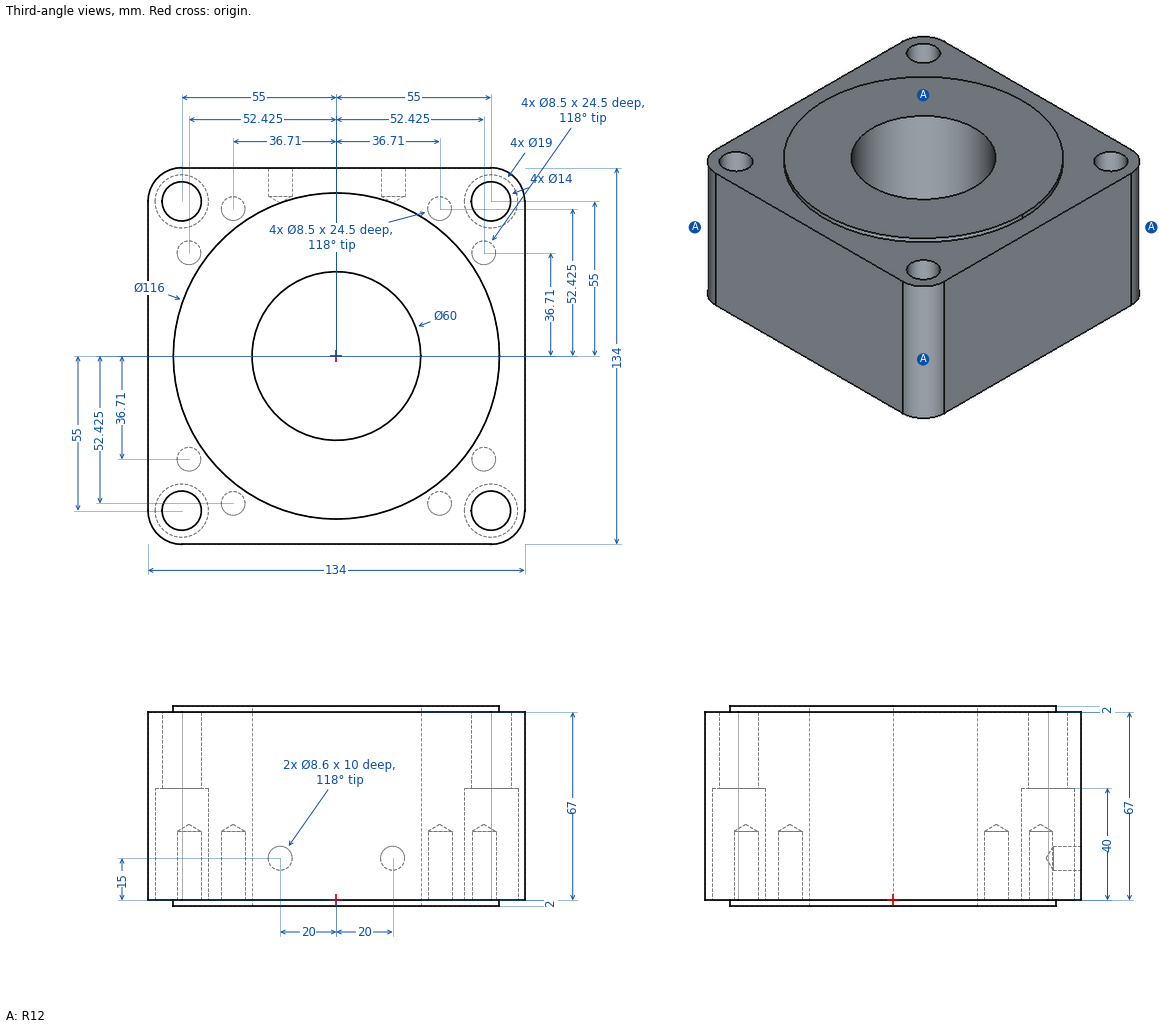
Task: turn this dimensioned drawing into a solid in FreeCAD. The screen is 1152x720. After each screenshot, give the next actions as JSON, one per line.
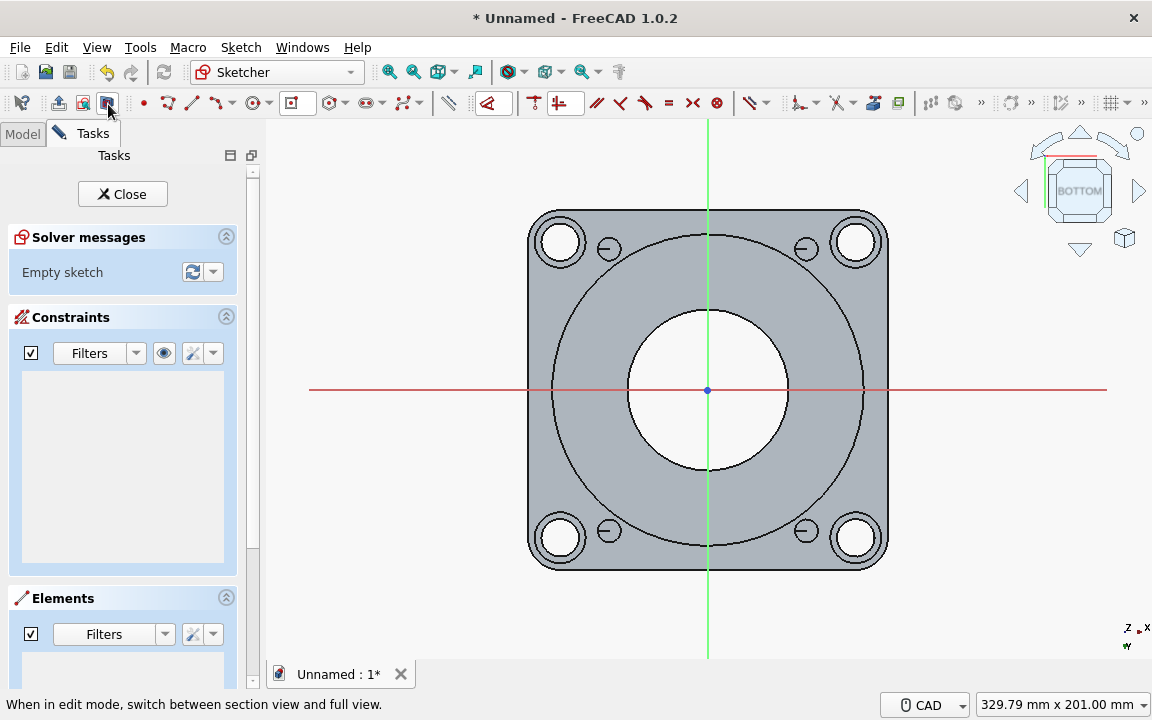
{"action": "scroll", "coordinate": [845, 392], "scroll_direction": "up", "scroll_amount": 2}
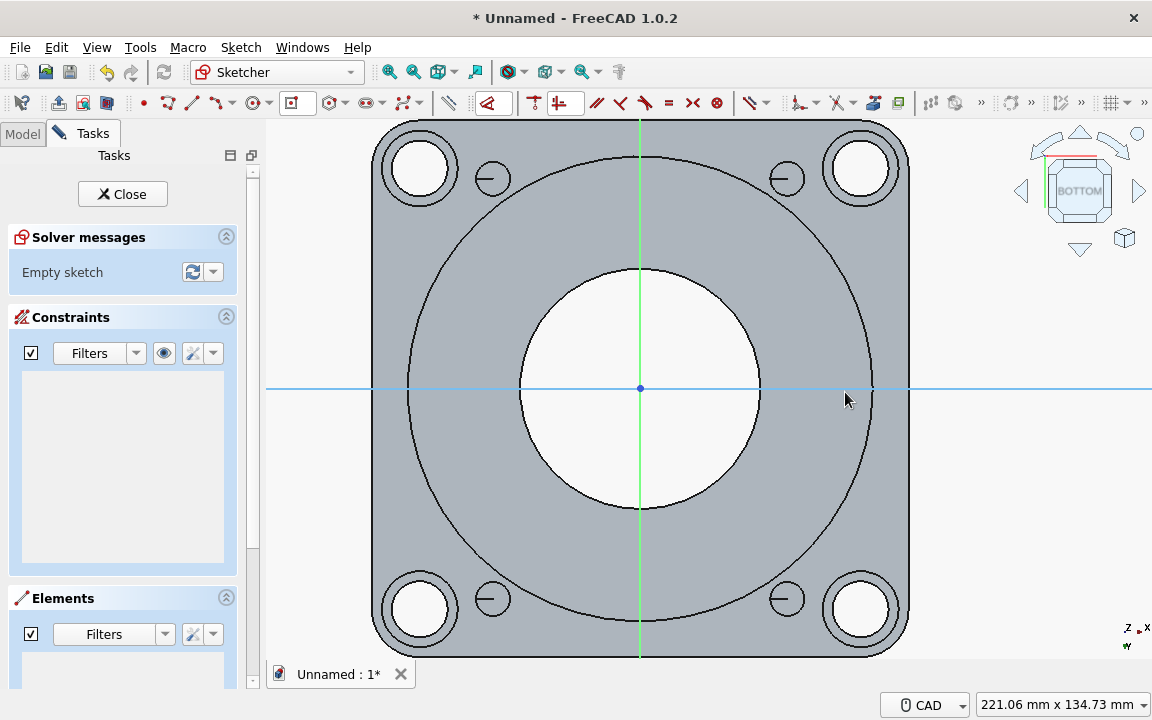
{"action": "left_click", "coordinate": [254, 104]}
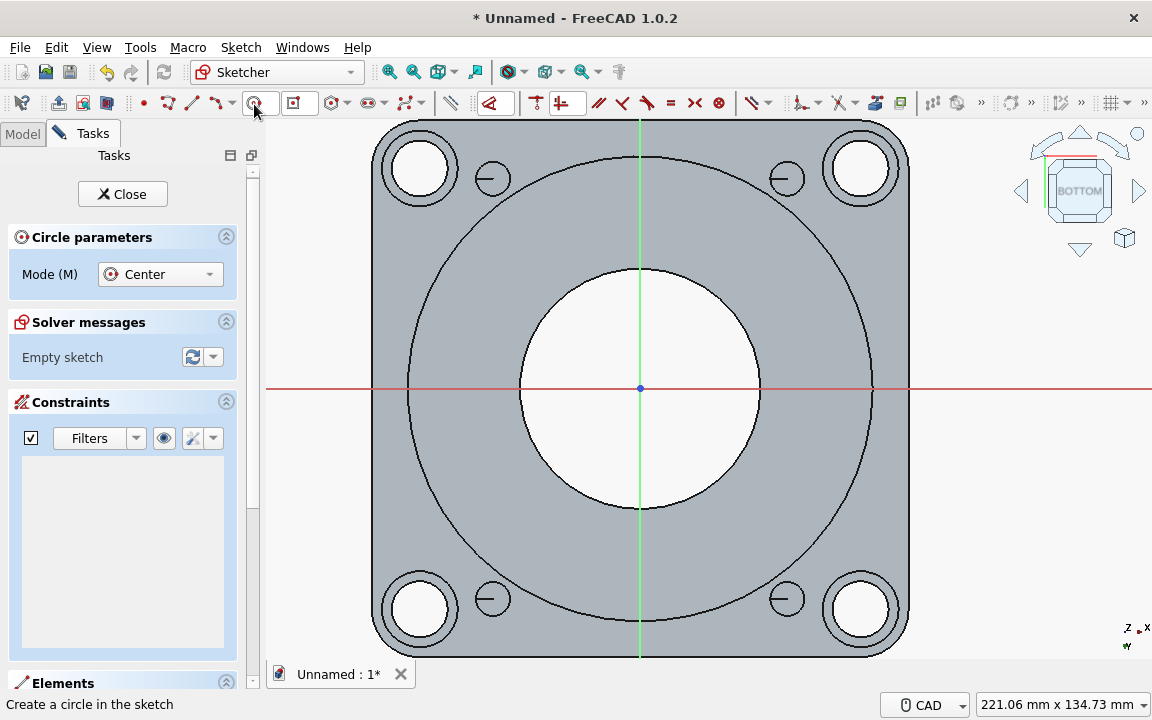
{"action": "scroll", "coordinate": [850, 536], "scroll_direction": "up", "scroll_amount": 2}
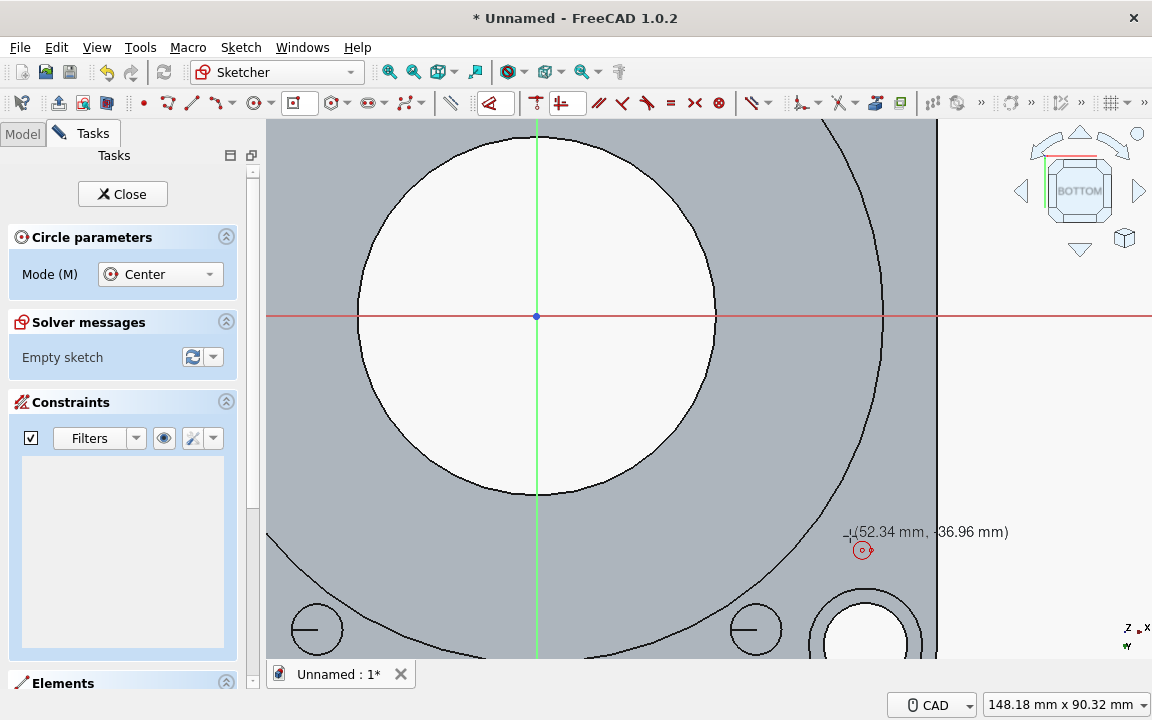
{"action": "left_click", "coordinate": [850, 536]}
{"action": "left_click", "coordinate": [868, 518]}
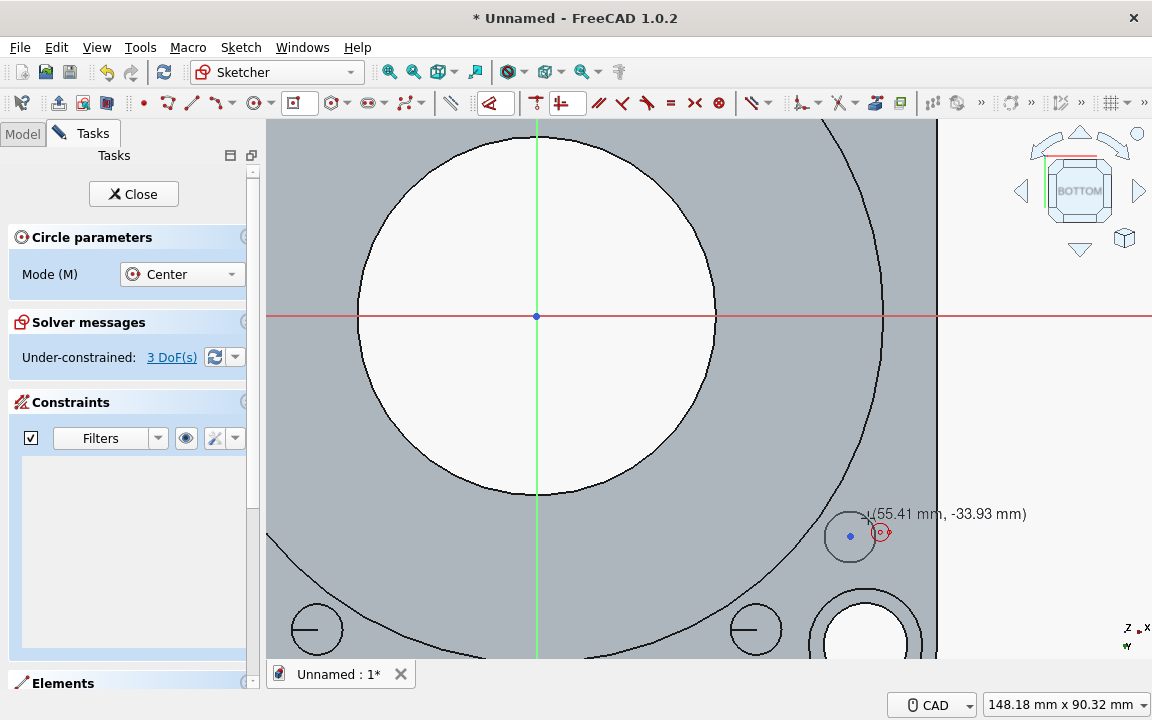
{"action": "scroll", "coordinate": [852, 537], "scroll_direction": "down", "scroll_amount": 2}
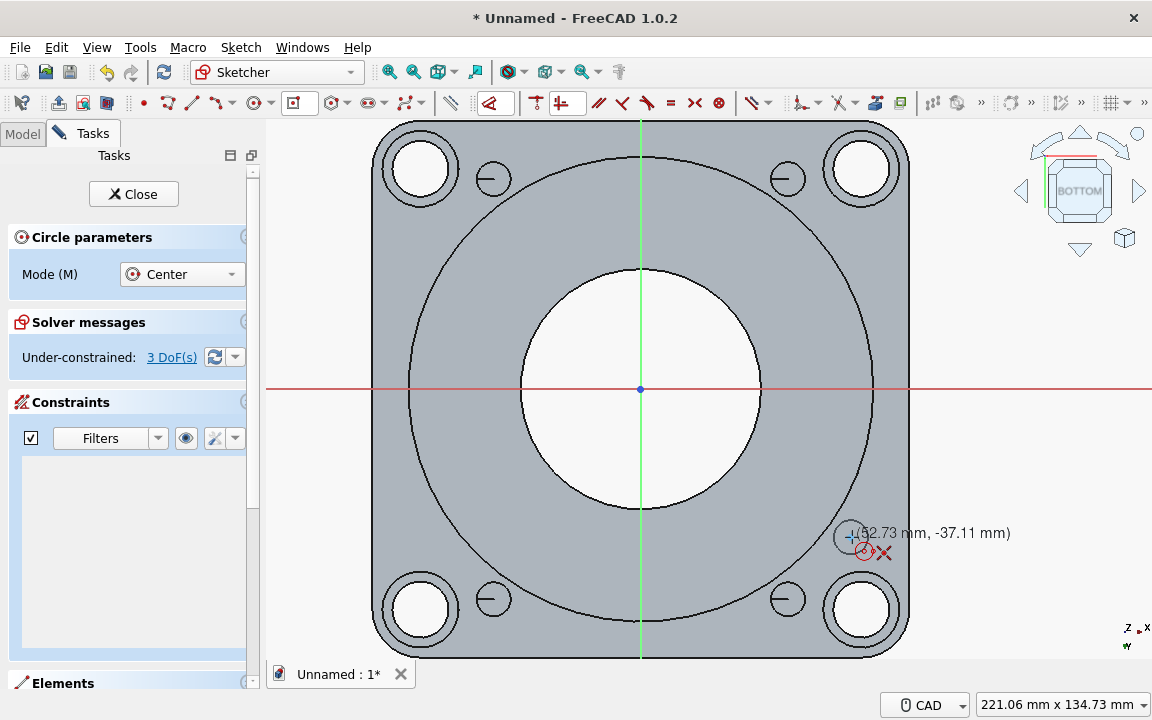
{"action": "scroll", "coordinate": [431, 536], "scroll_direction": "up", "scroll_amount": 2}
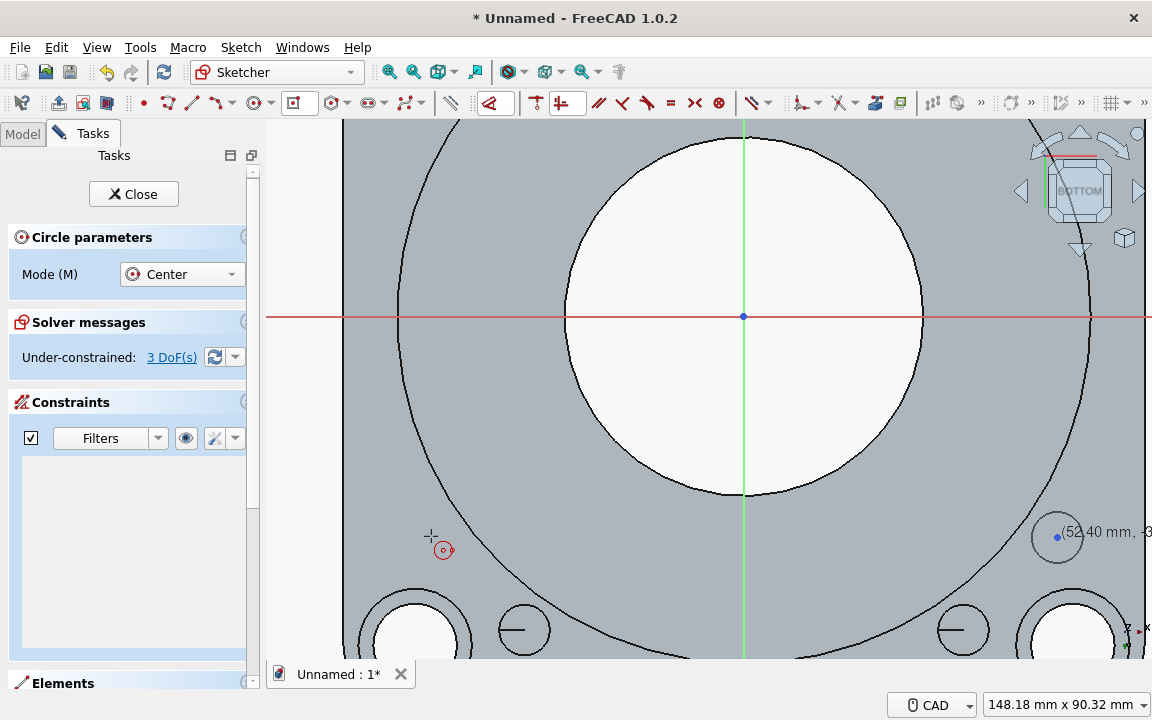
{"action": "left_click", "coordinate": [431, 536]}
{"action": "left_click", "coordinate": [449, 518]}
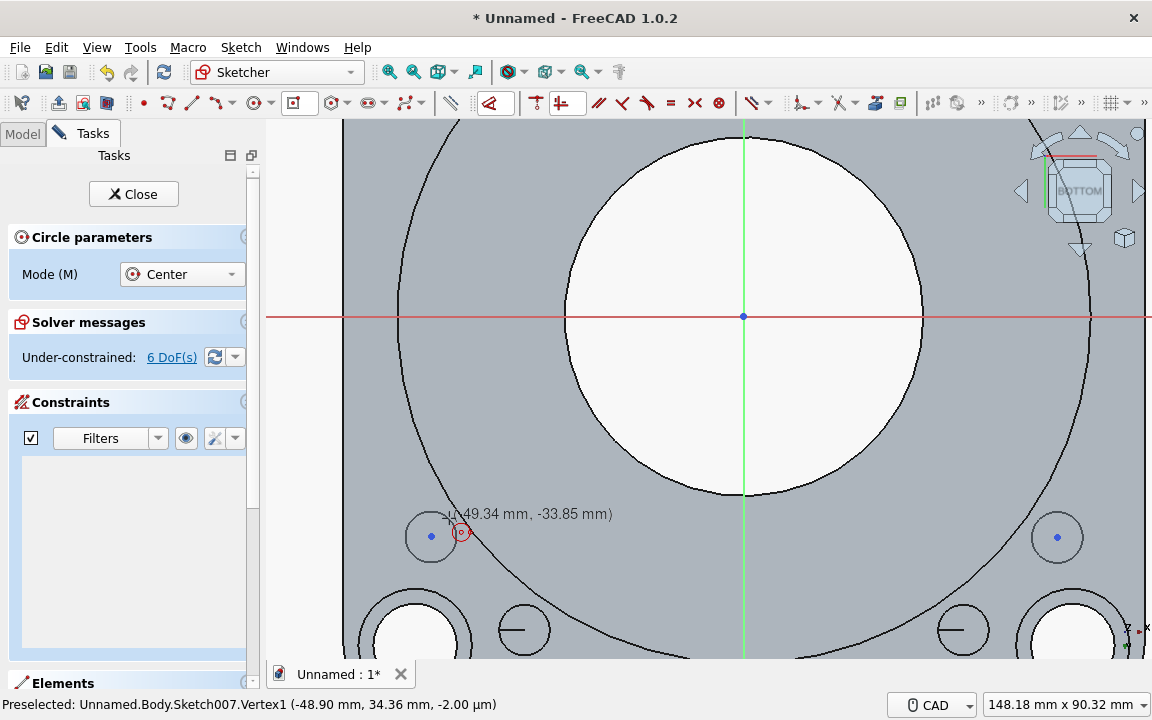
{"action": "scroll", "coordinate": [430, 536], "scroll_direction": "down", "scroll_amount": 2}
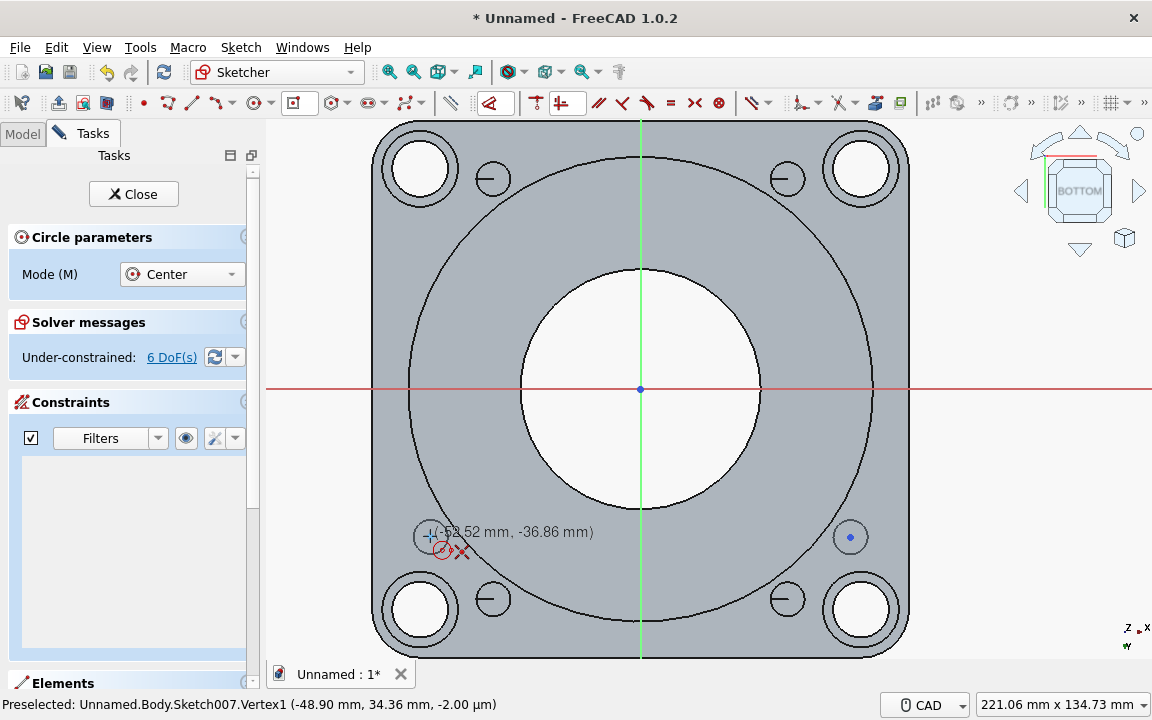
{"action": "scroll", "coordinate": [430, 242], "scroll_direction": "up", "scroll_amount": 2}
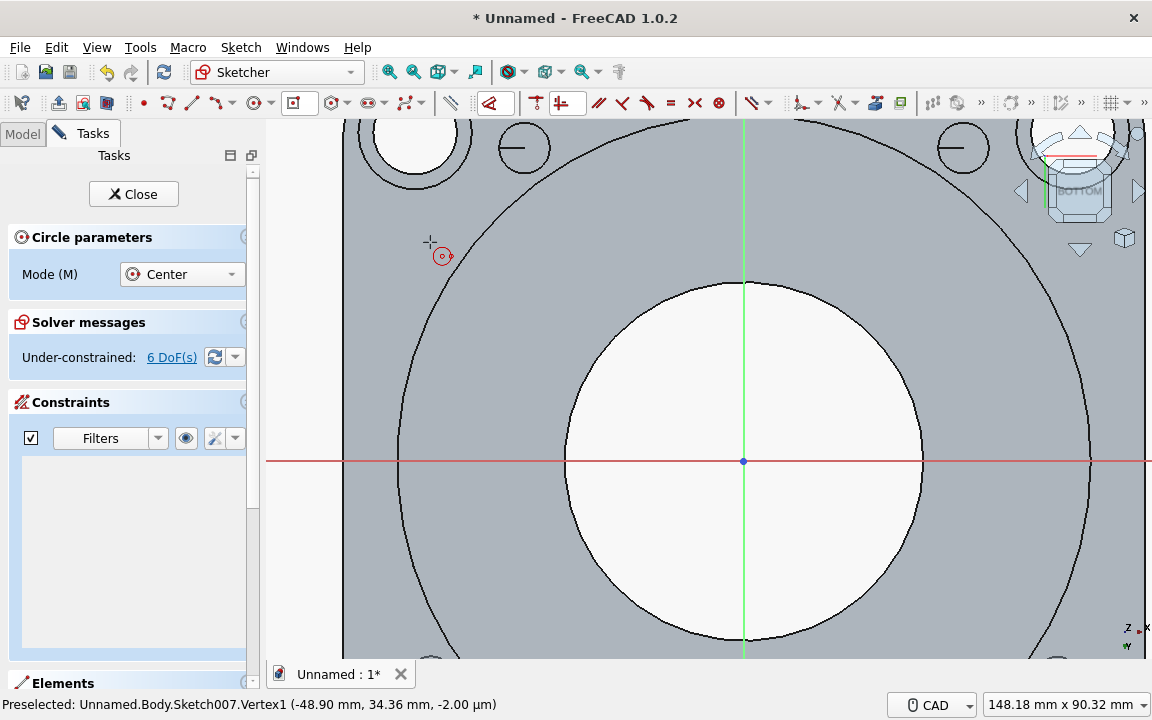
{"action": "left_click", "coordinate": [431, 242]}
{"action": "left_click", "coordinate": [449, 224]}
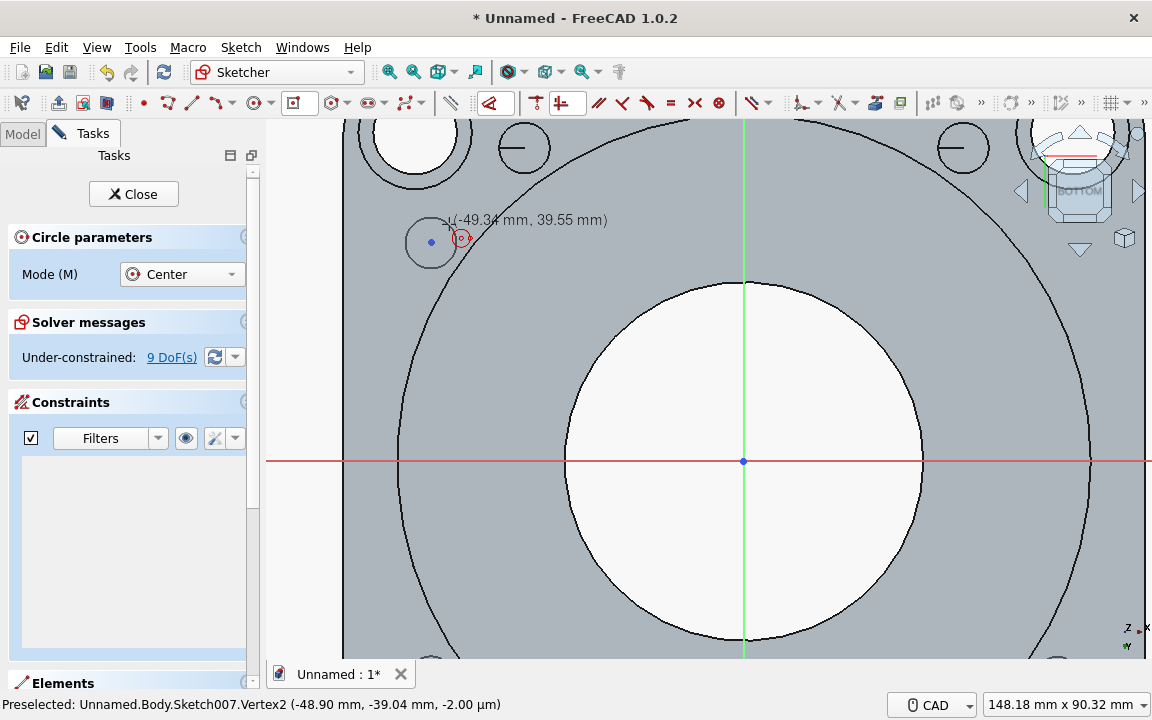
{"action": "scroll", "coordinate": [430, 242], "scroll_direction": "down", "scroll_amount": 2}